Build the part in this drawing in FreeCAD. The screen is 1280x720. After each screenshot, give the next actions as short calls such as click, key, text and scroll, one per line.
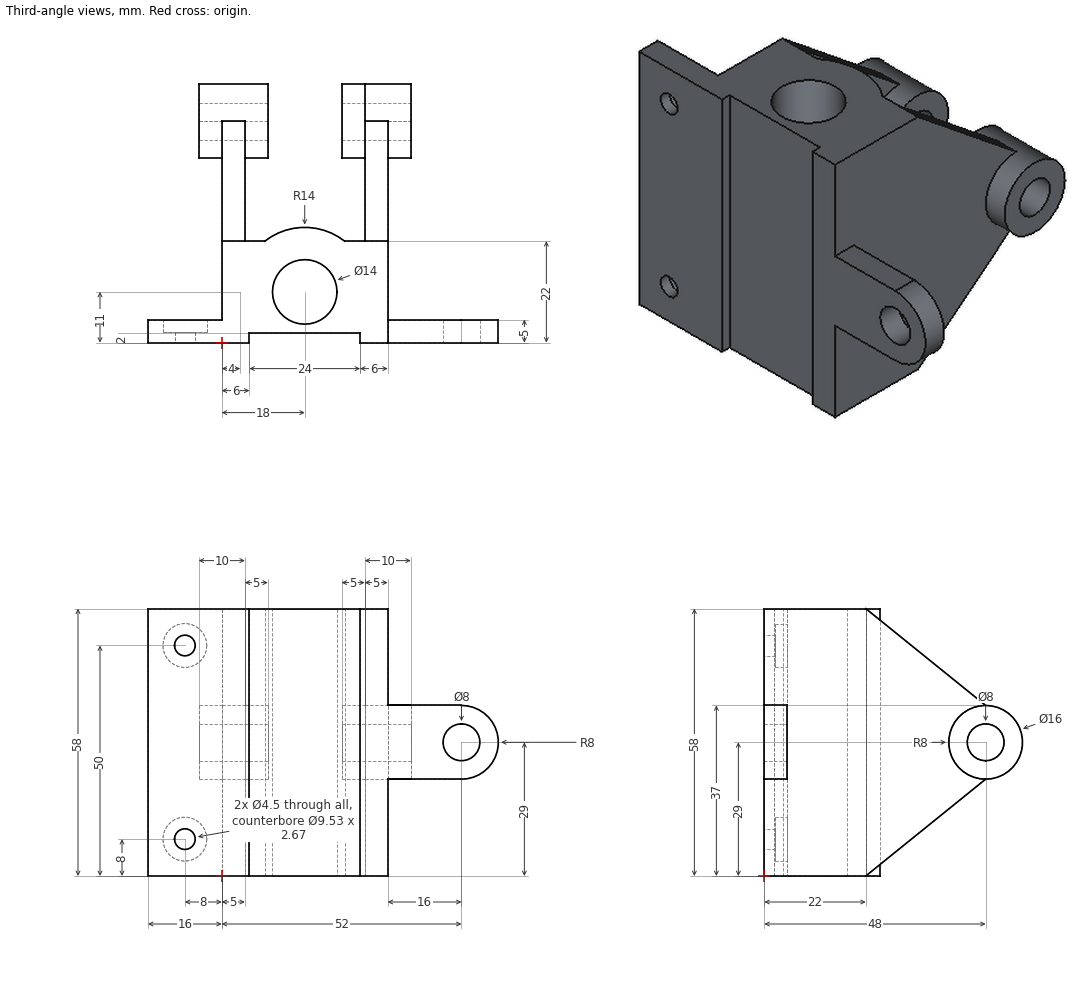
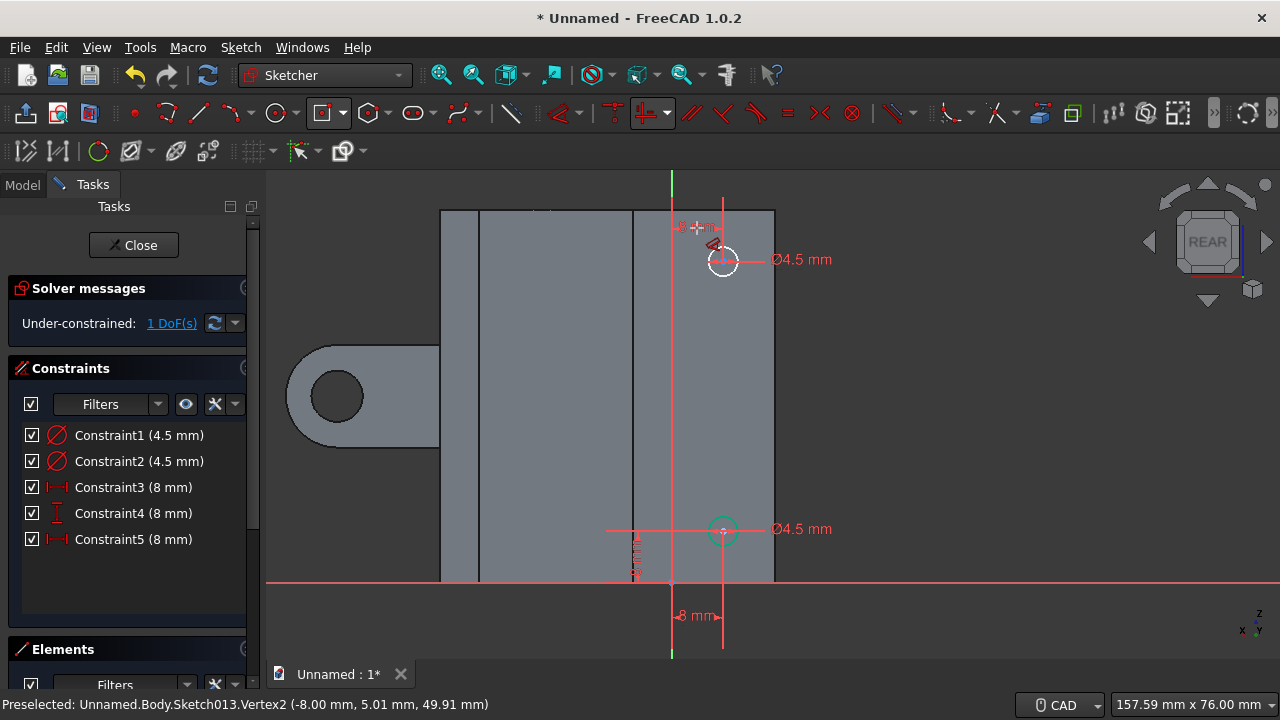
click(723, 262)
click(638, 422)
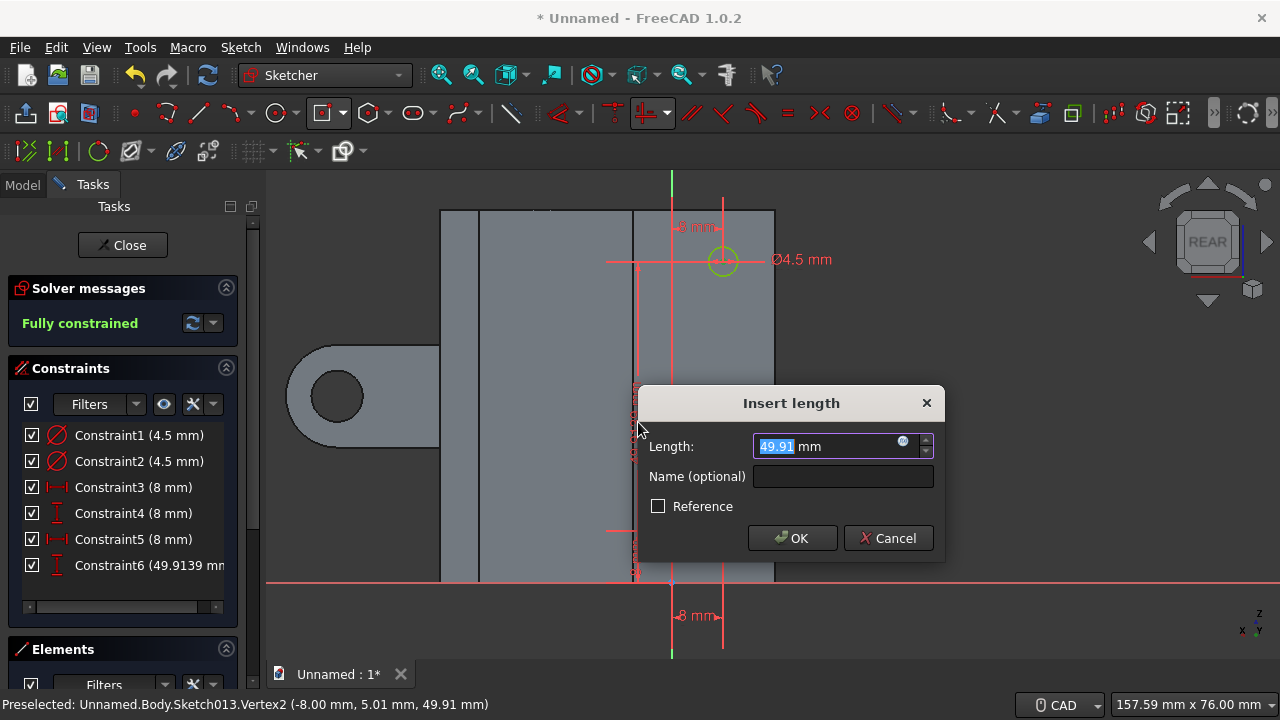
text(50)
key(Return)
key(Escape)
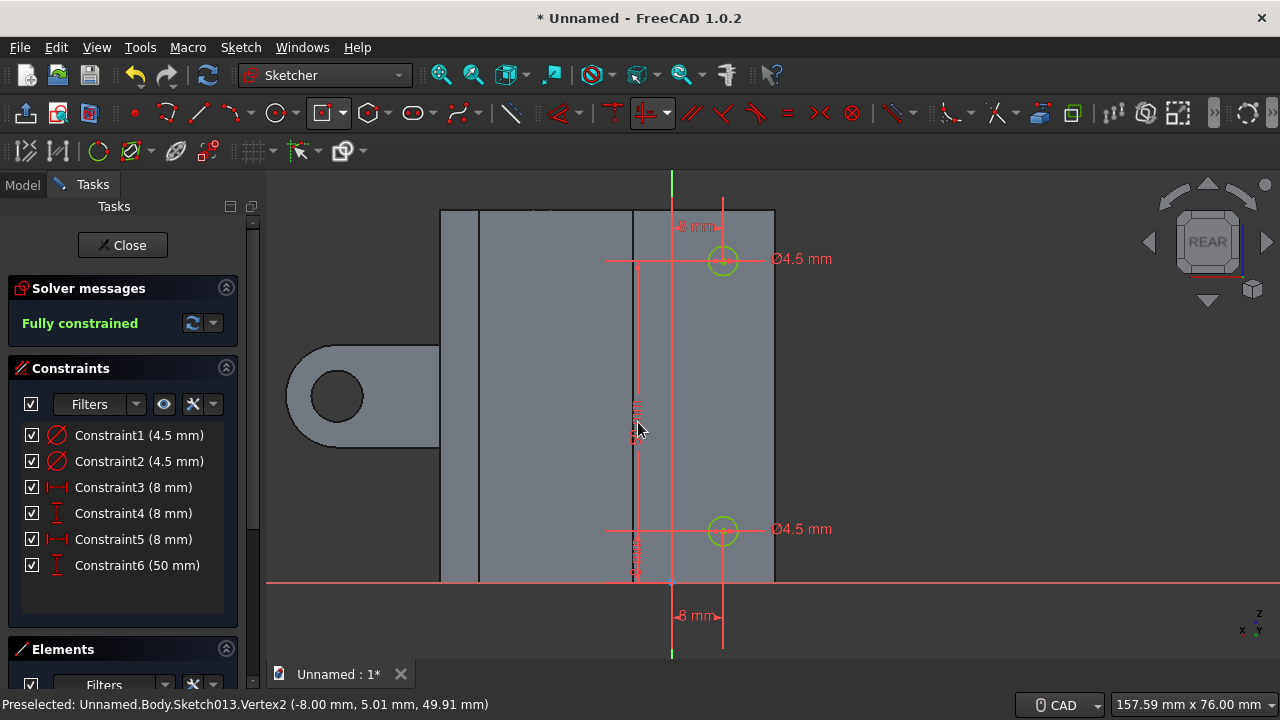
click(123, 245)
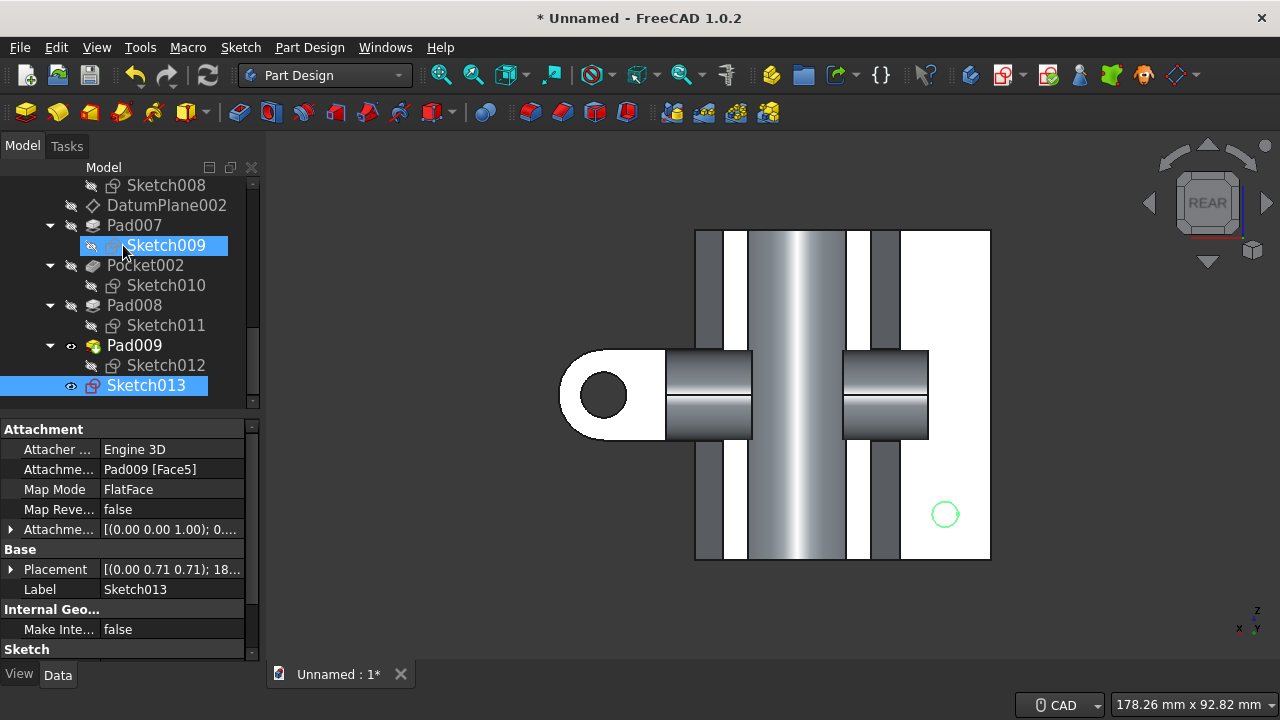
click(272, 112)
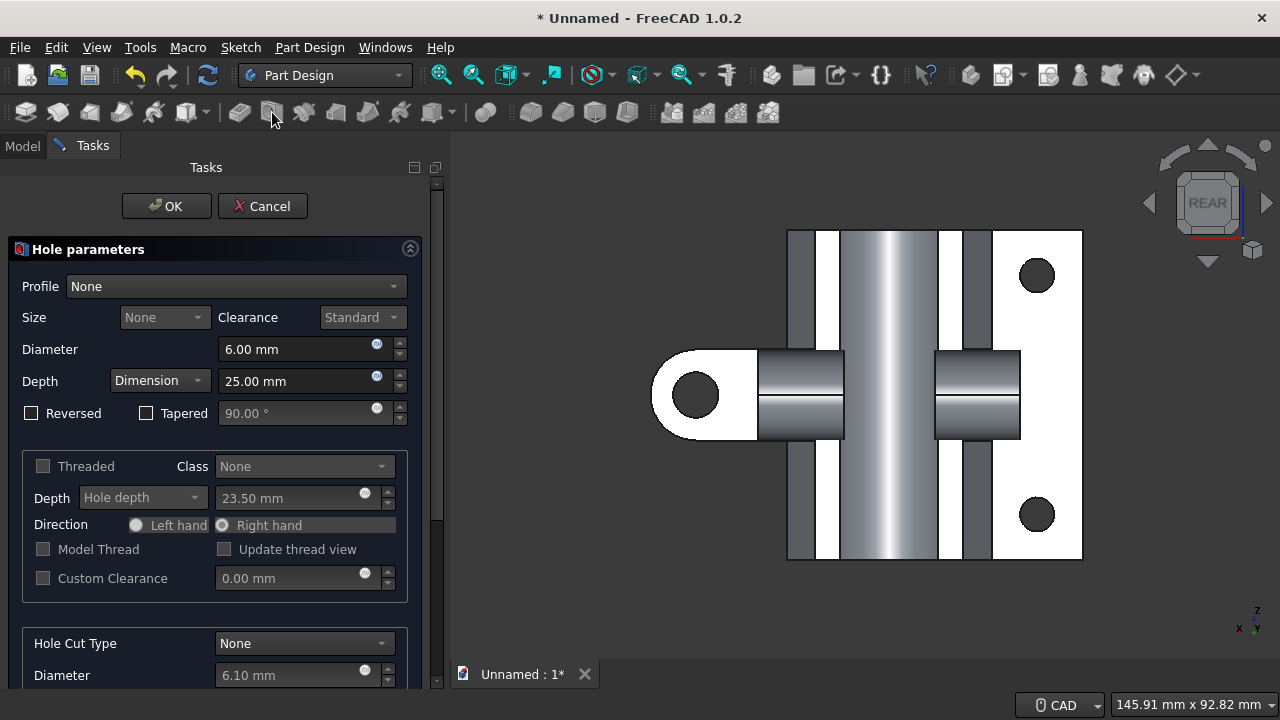
triple_click(305, 349)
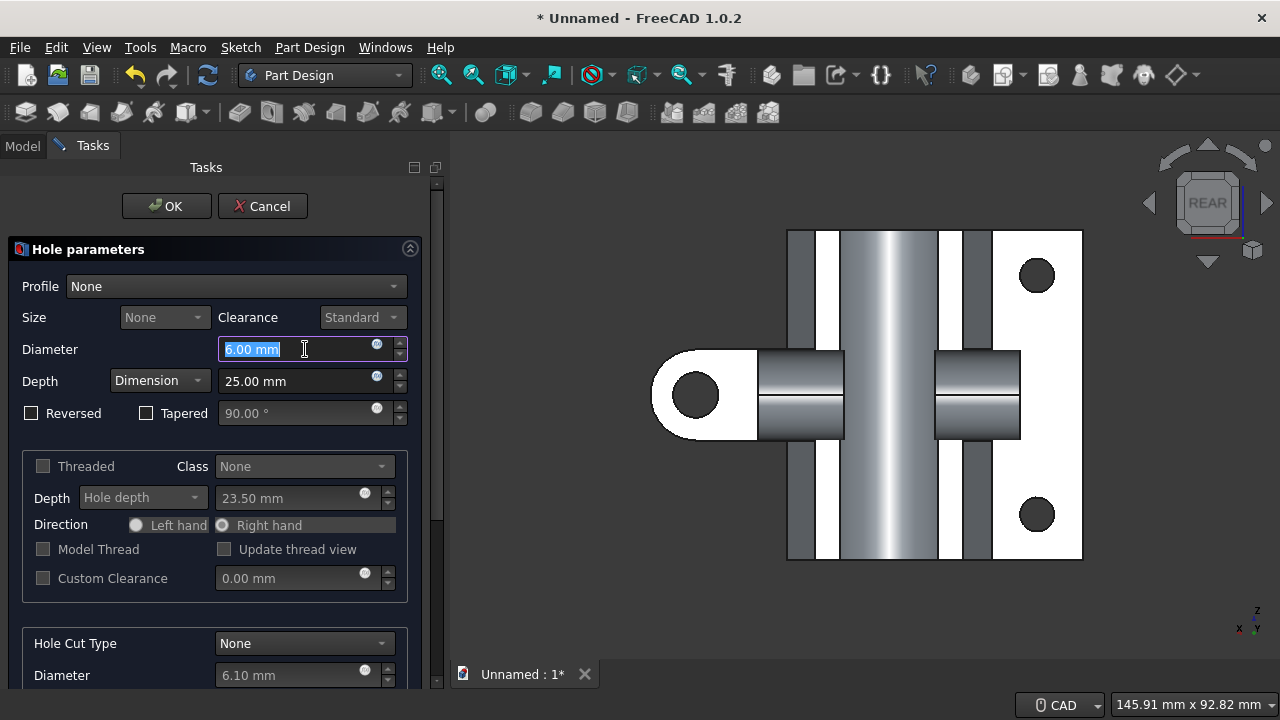
text(4.5)
key(Tab)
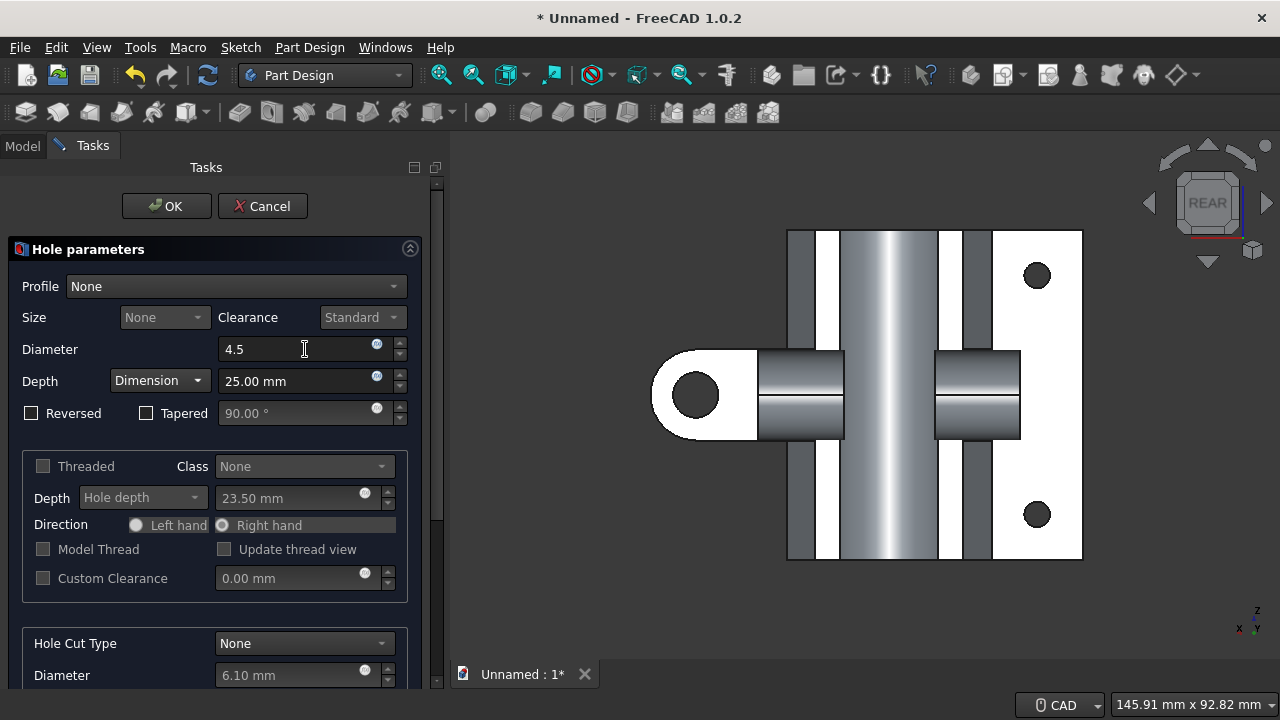
click(161, 380)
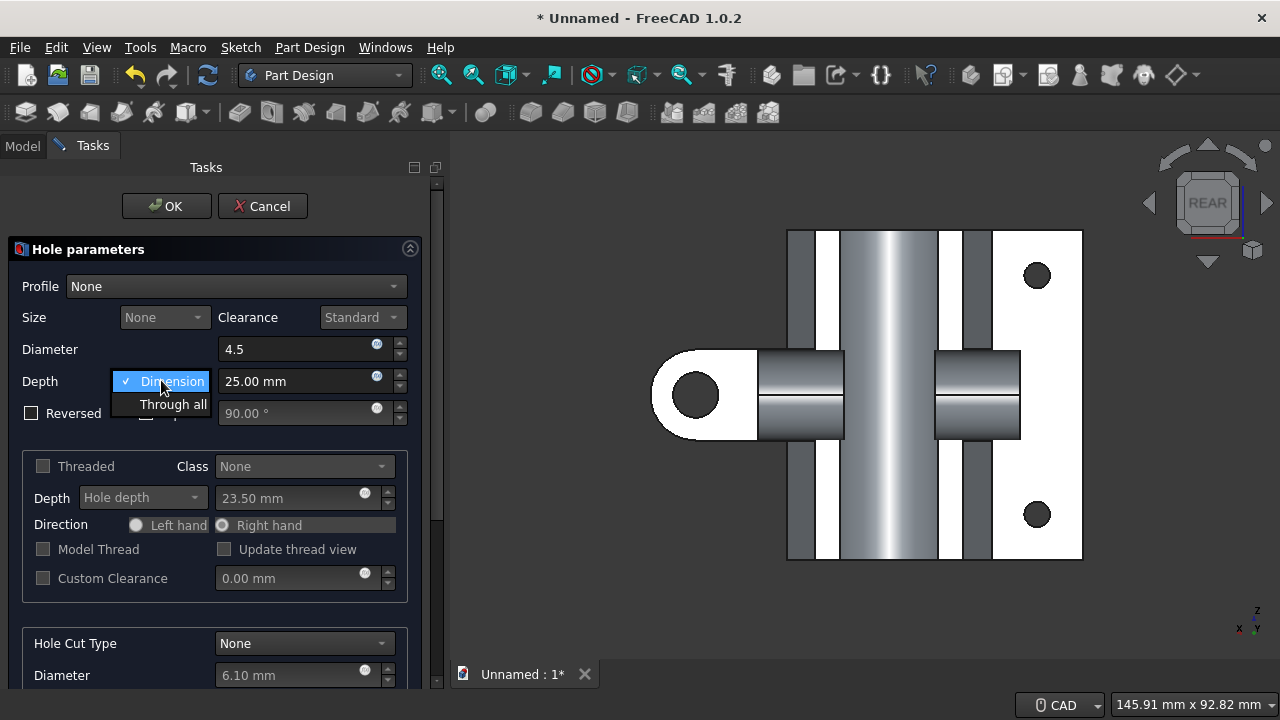
click(160, 404)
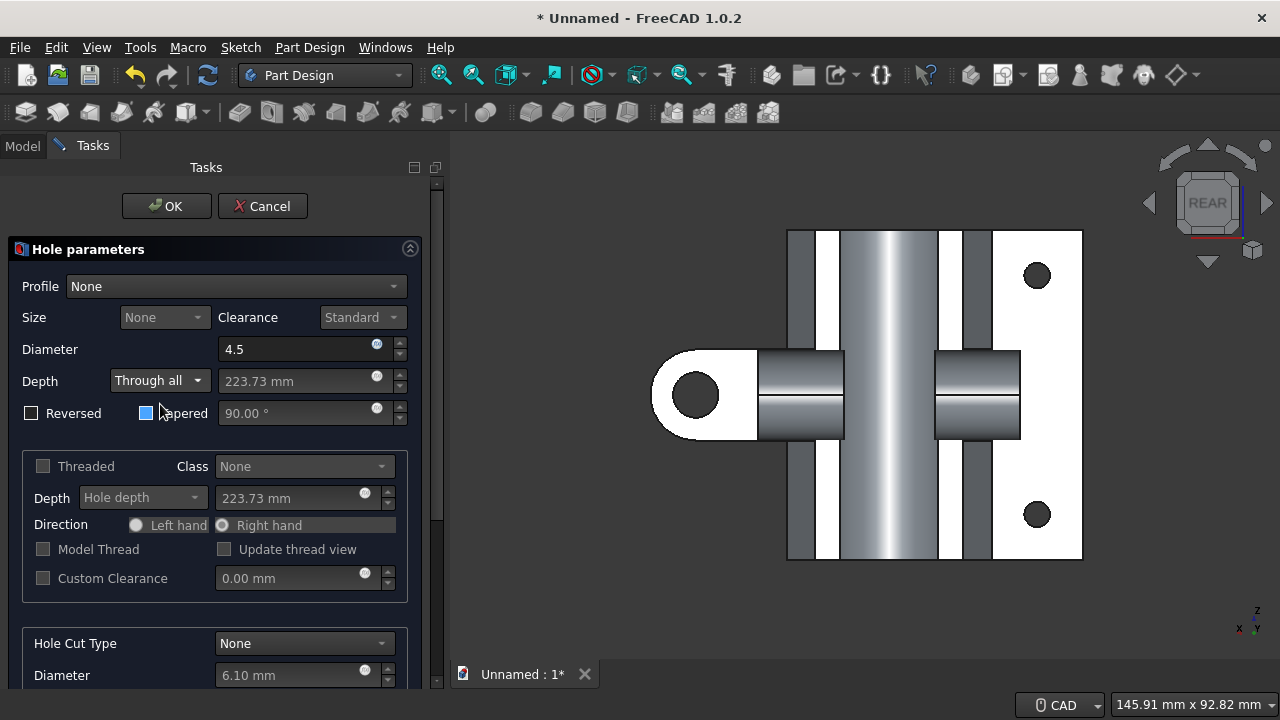
click(306, 644)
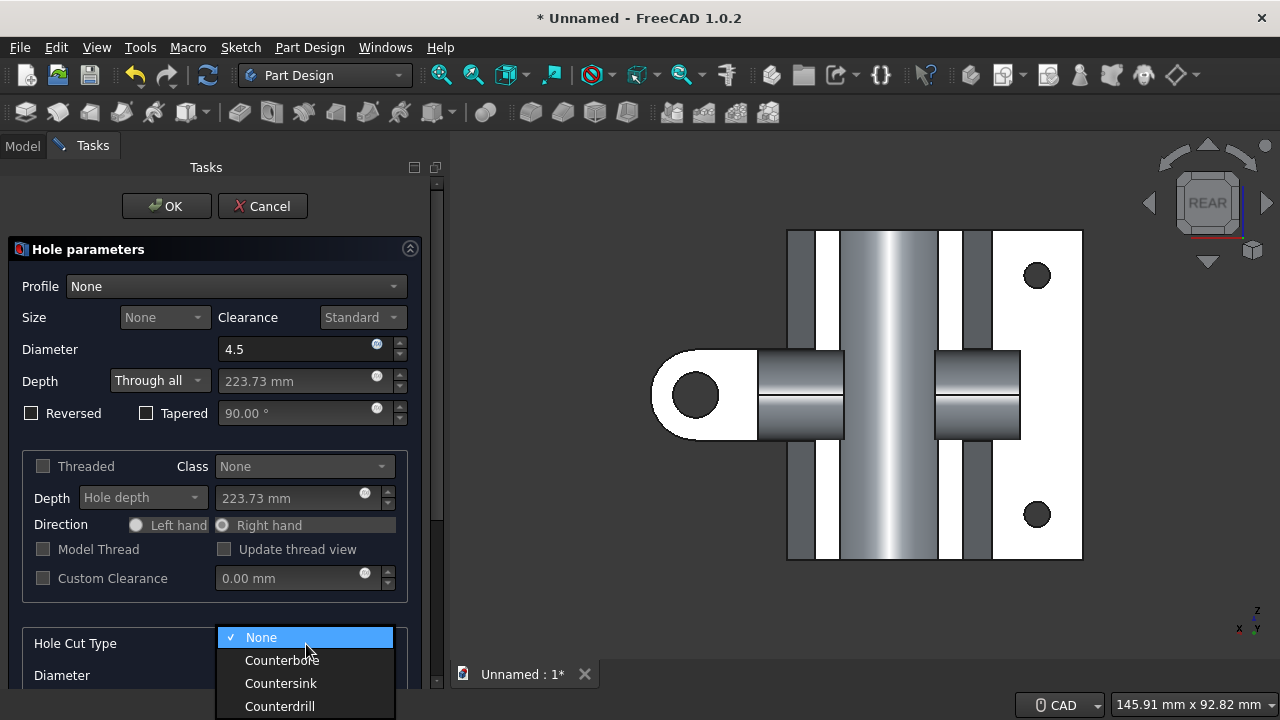
click(304, 660)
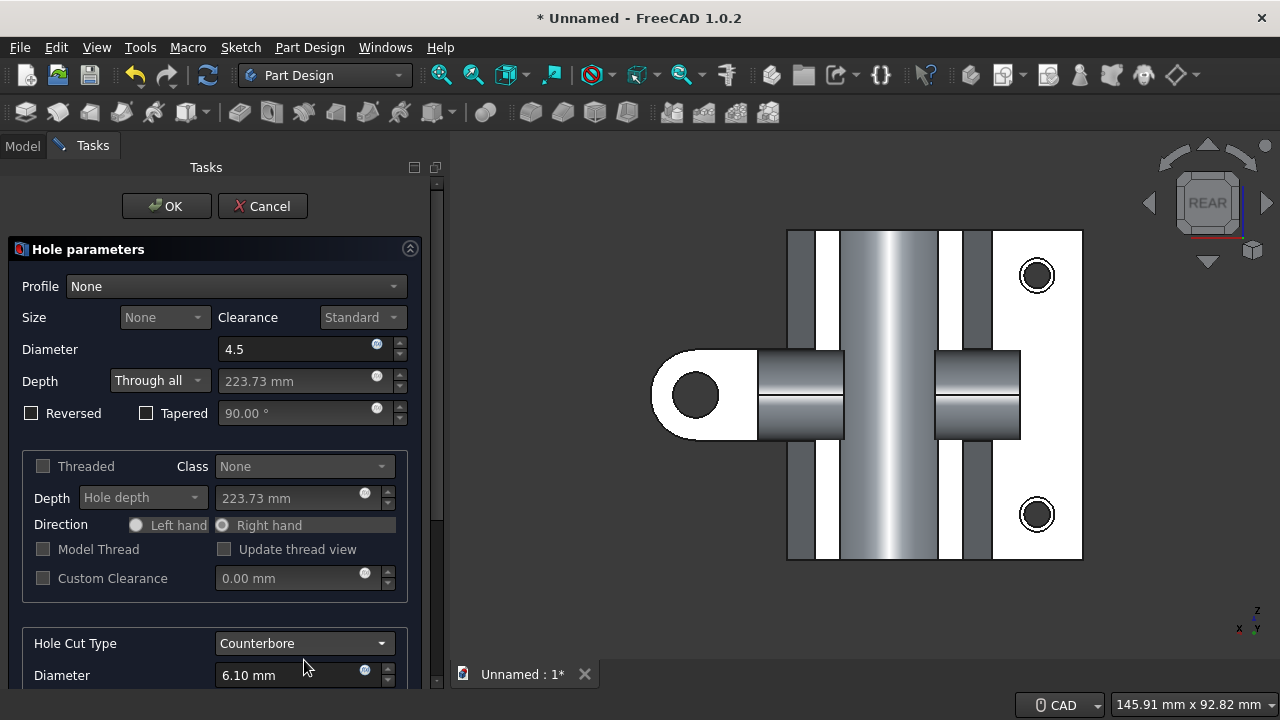
triple_click(298, 675)